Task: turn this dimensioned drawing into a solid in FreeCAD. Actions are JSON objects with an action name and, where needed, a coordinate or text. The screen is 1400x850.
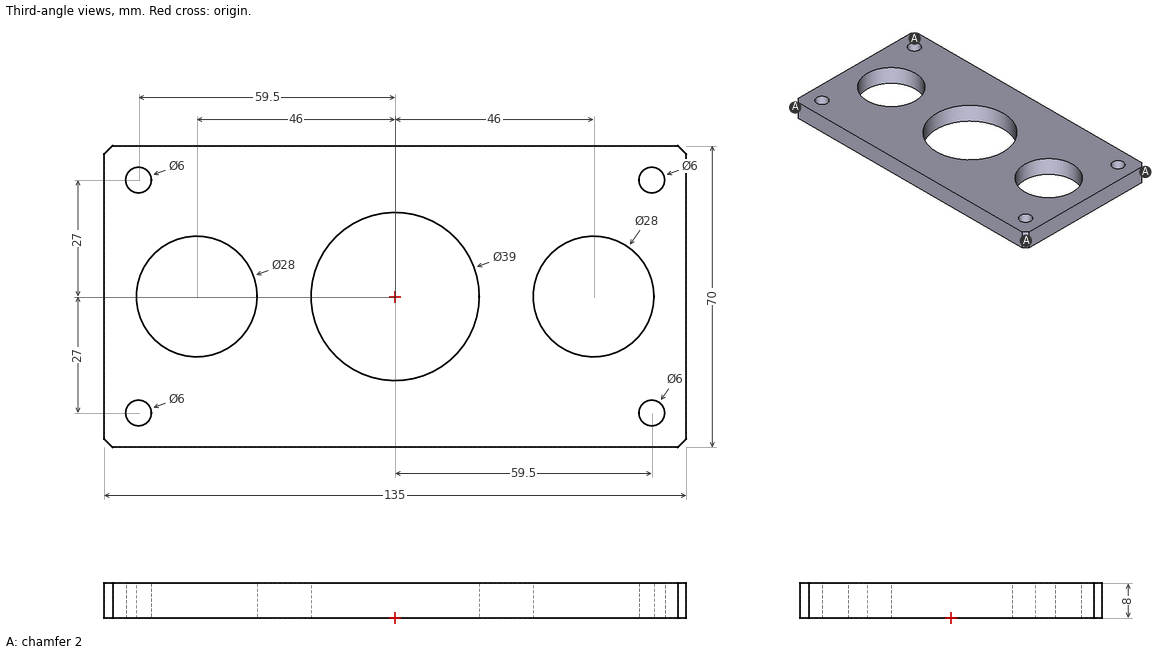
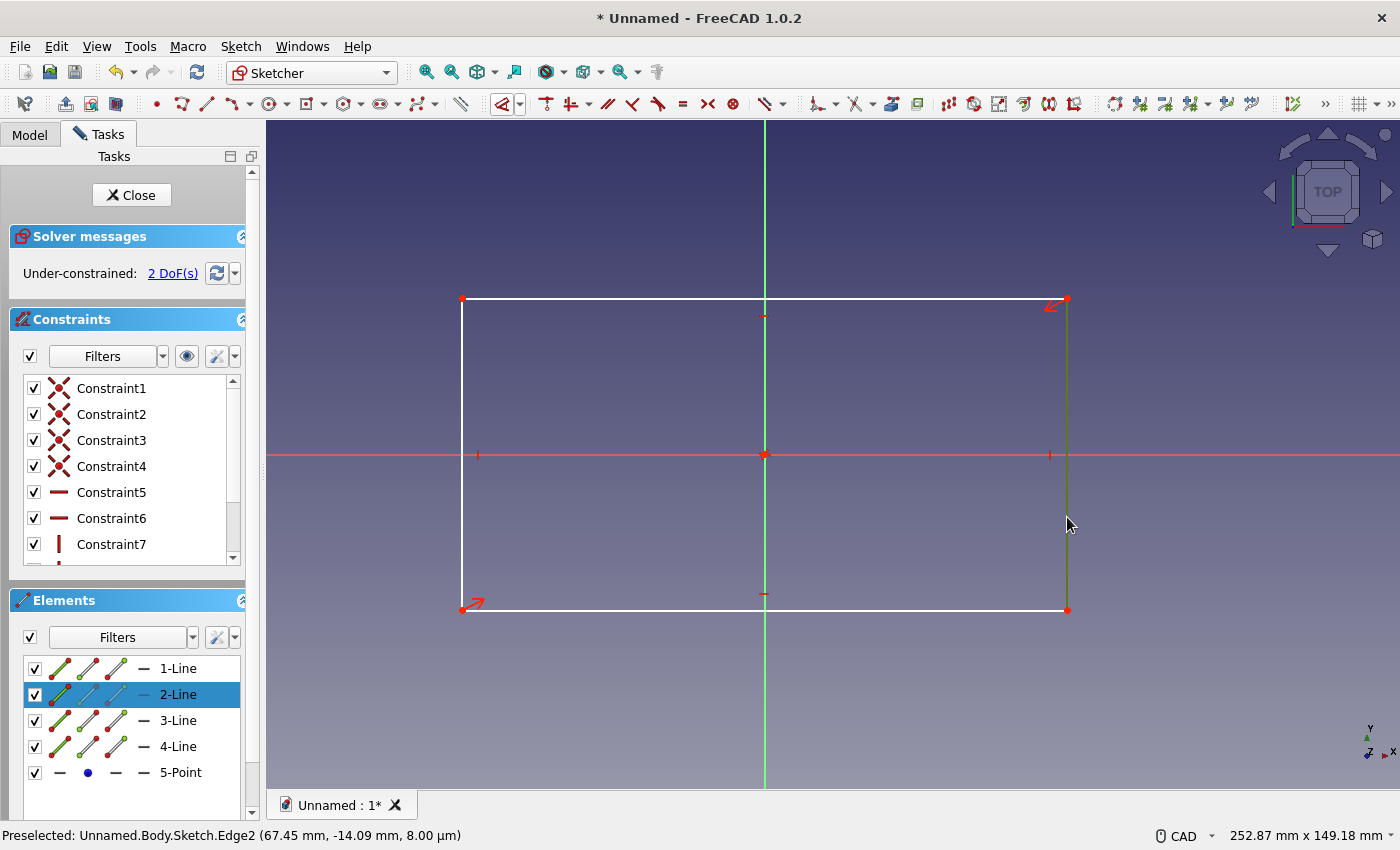
{"action": "key", "text": "i"}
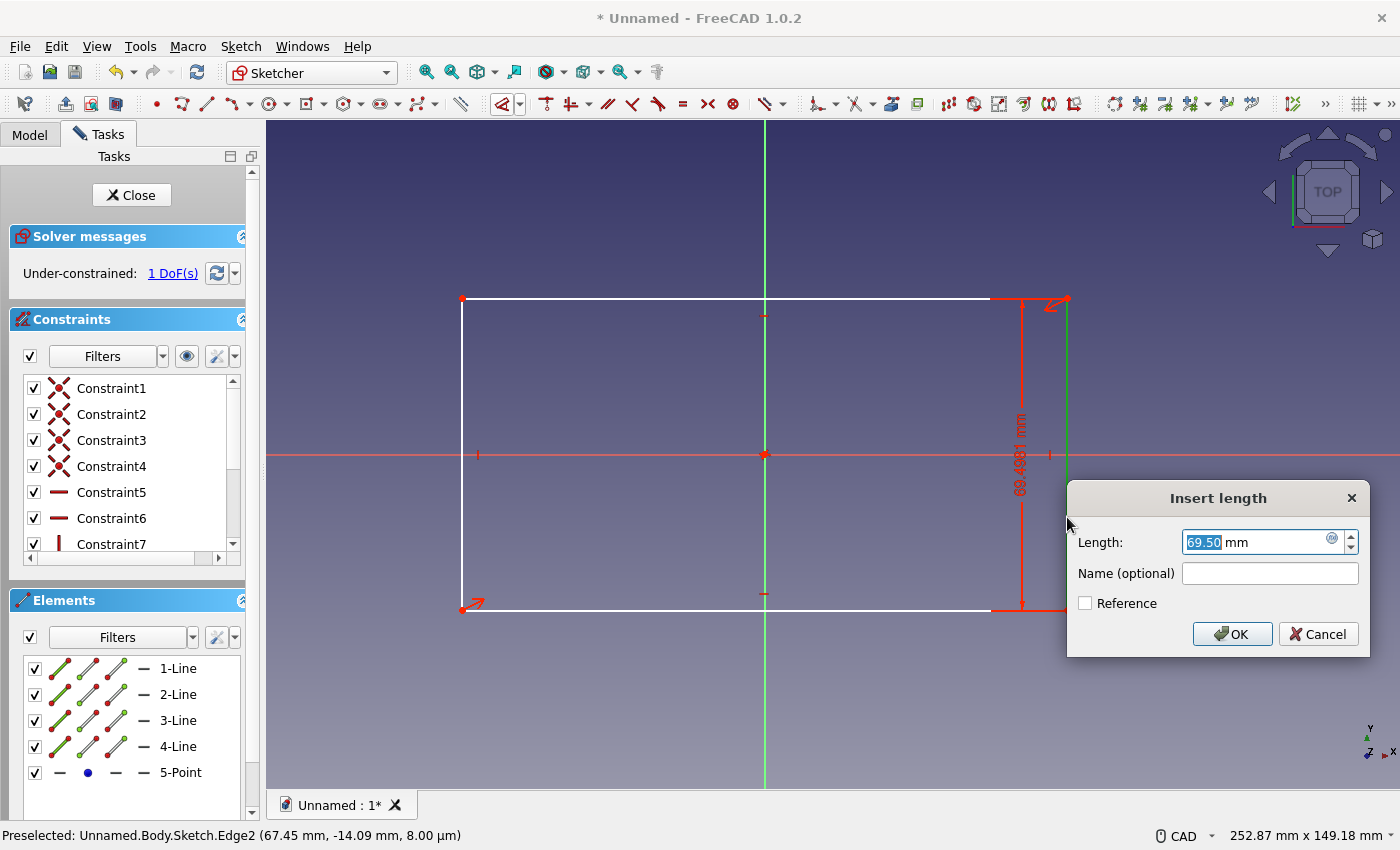
{"action": "type", "text": "70"}
{"action": "key", "text": "Return"}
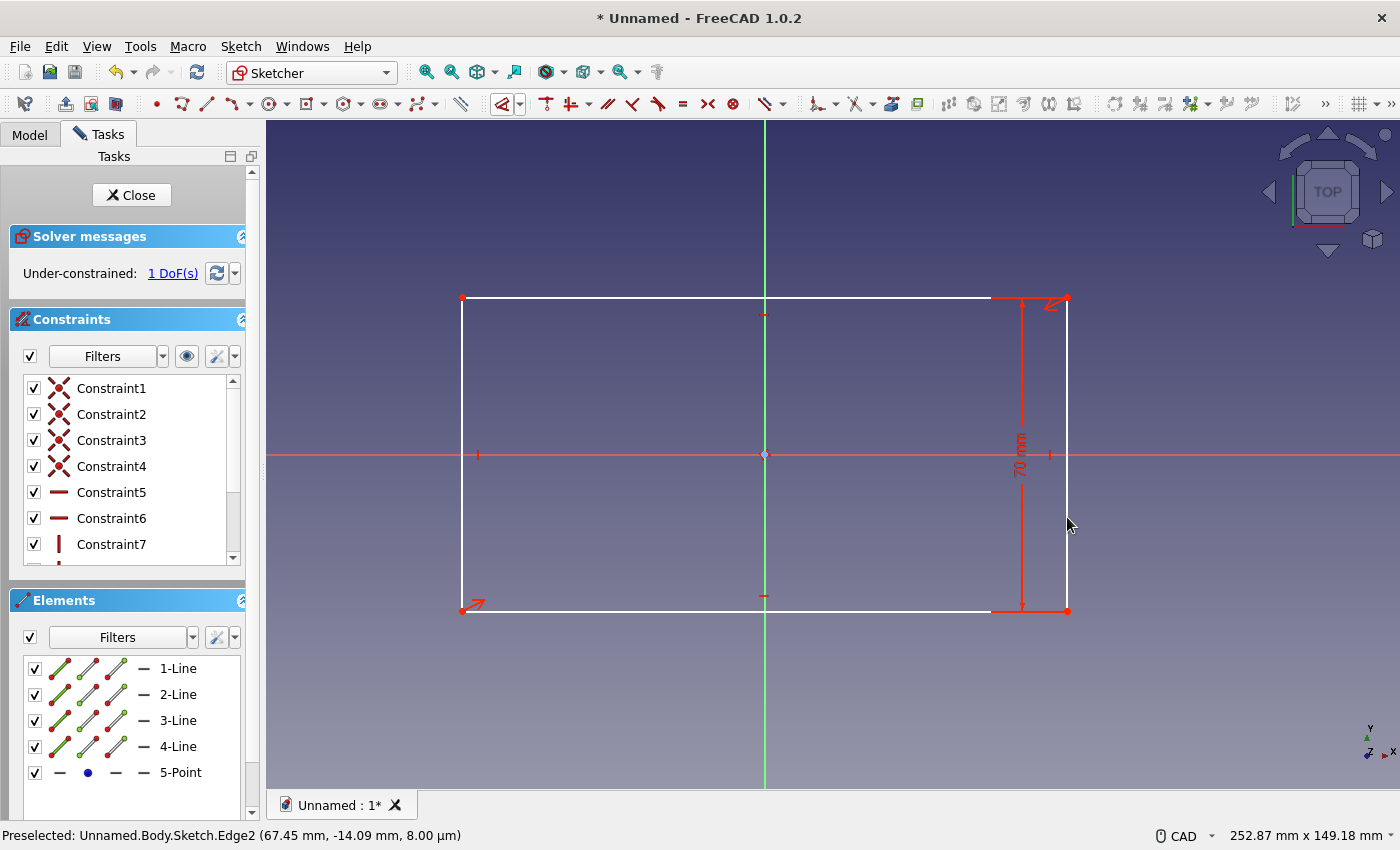
{"action": "left_click", "coordinate": [644, 612]}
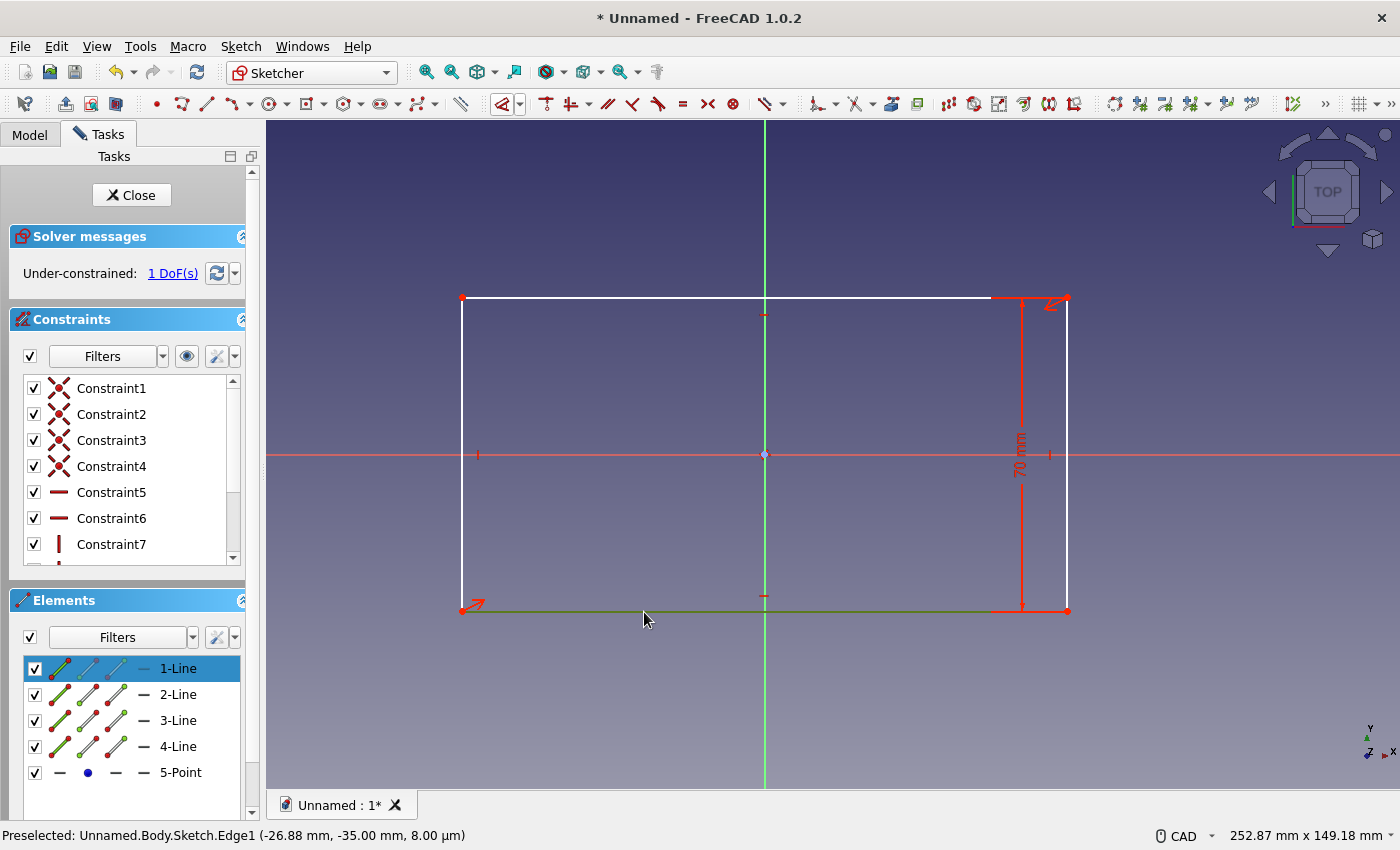
{"action": "key", "text": "l"}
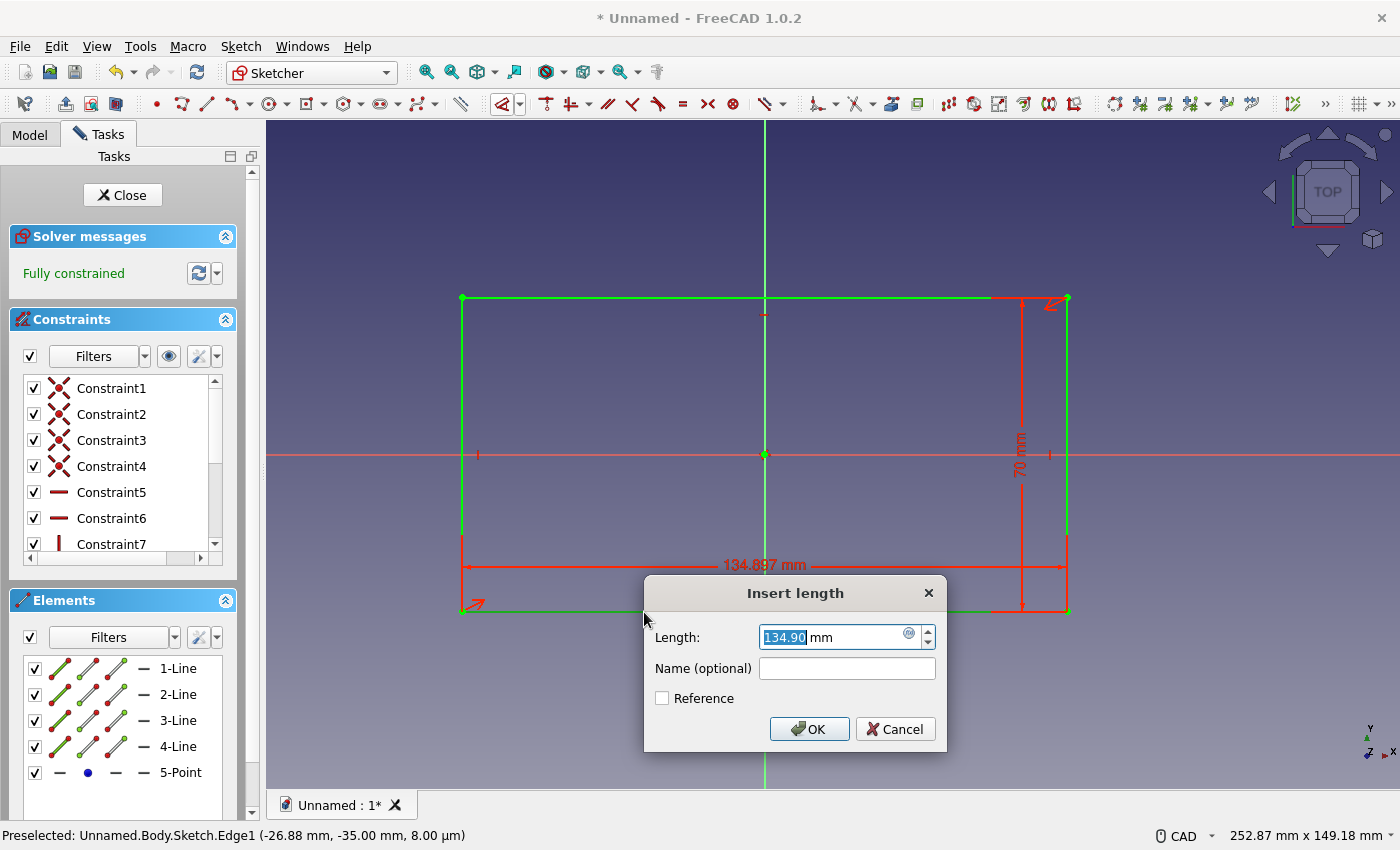
{"action": "type", "text": "135"}
{"action": "key", "text": "Return"}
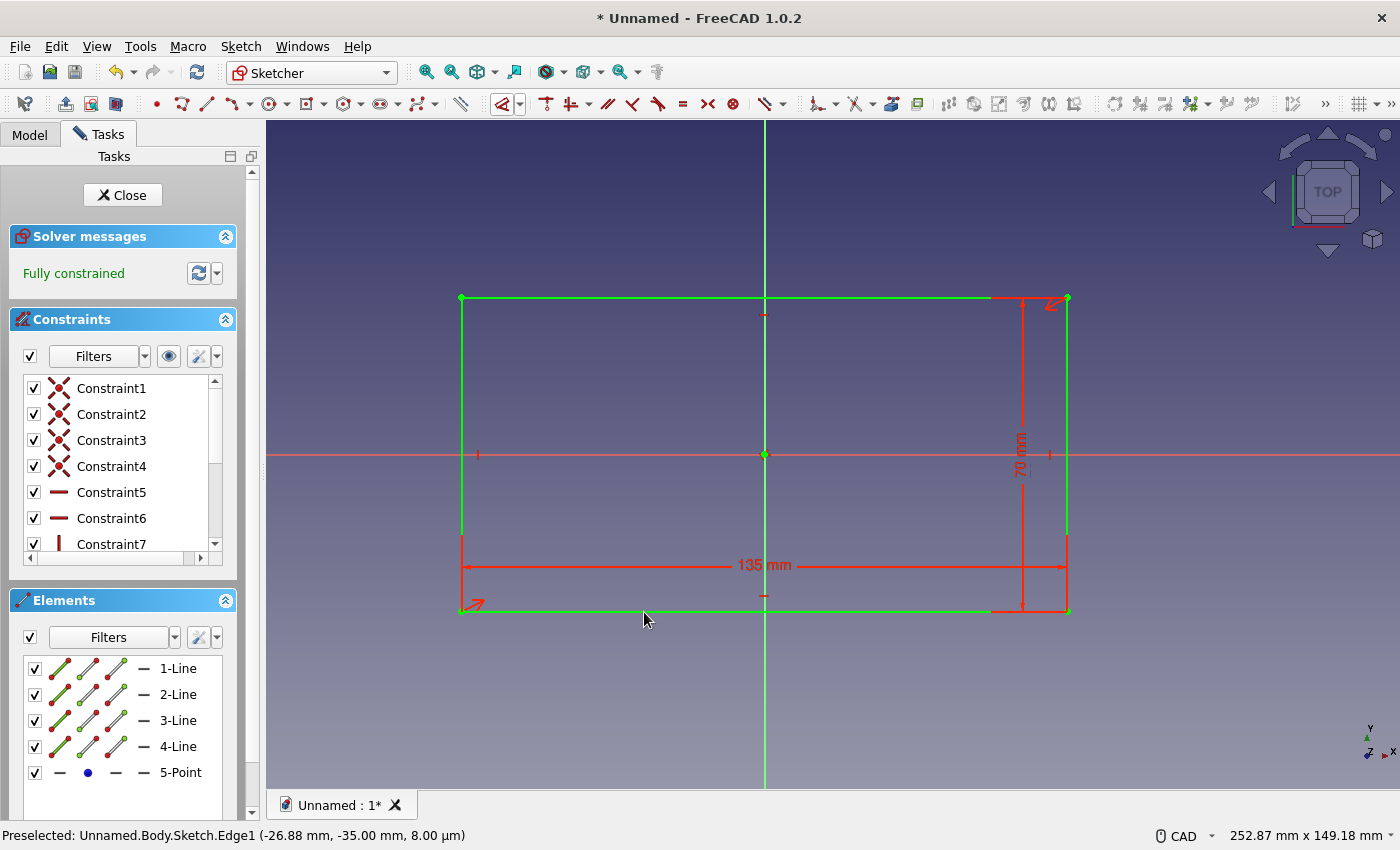
{"action": "left_click", "coordinate": [123, 195]}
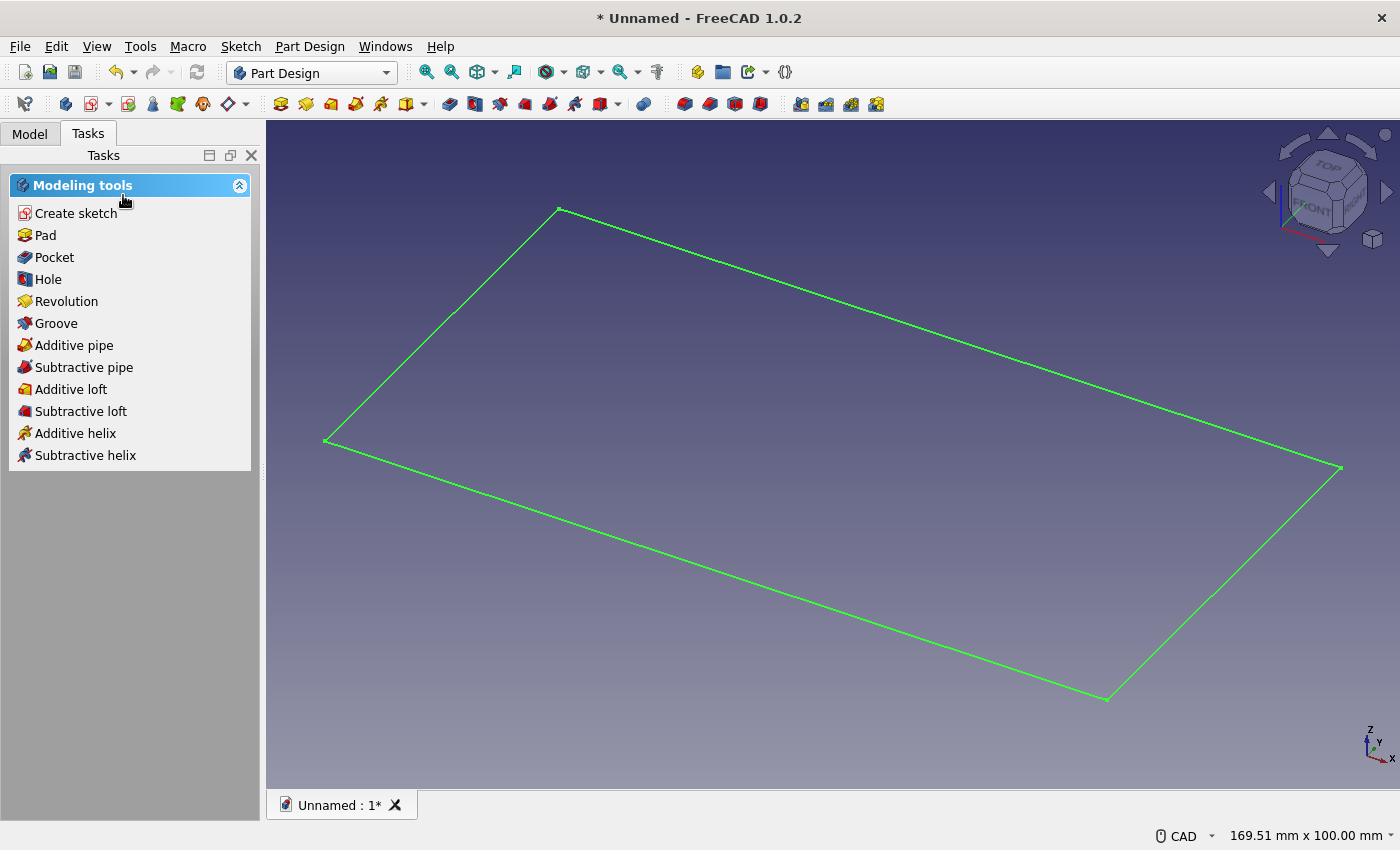
{"action": "left_click", "coordinate": [281, 104]}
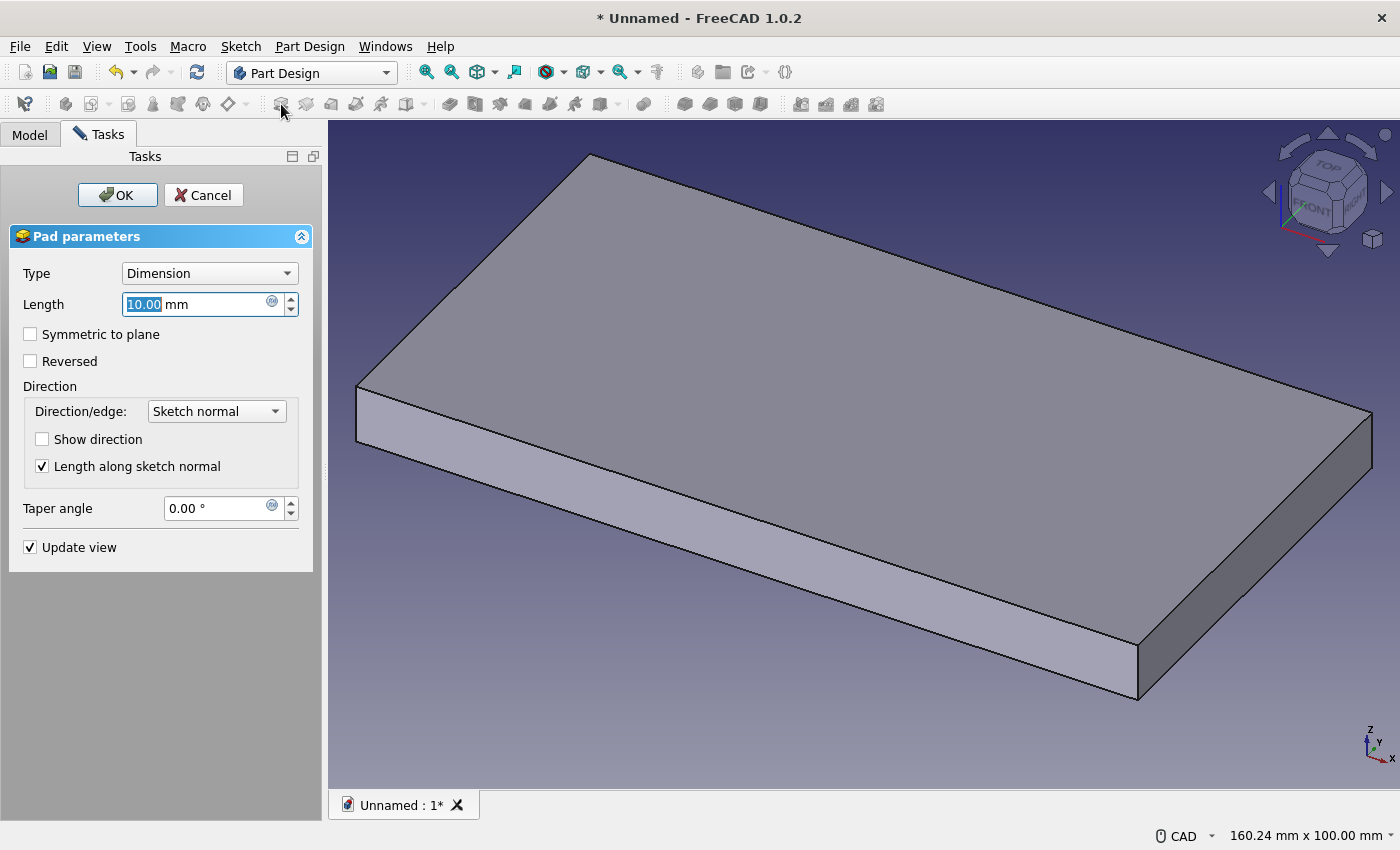
{"action": "type", "text": "8"}
{"action": "key", "text": "Tab"}